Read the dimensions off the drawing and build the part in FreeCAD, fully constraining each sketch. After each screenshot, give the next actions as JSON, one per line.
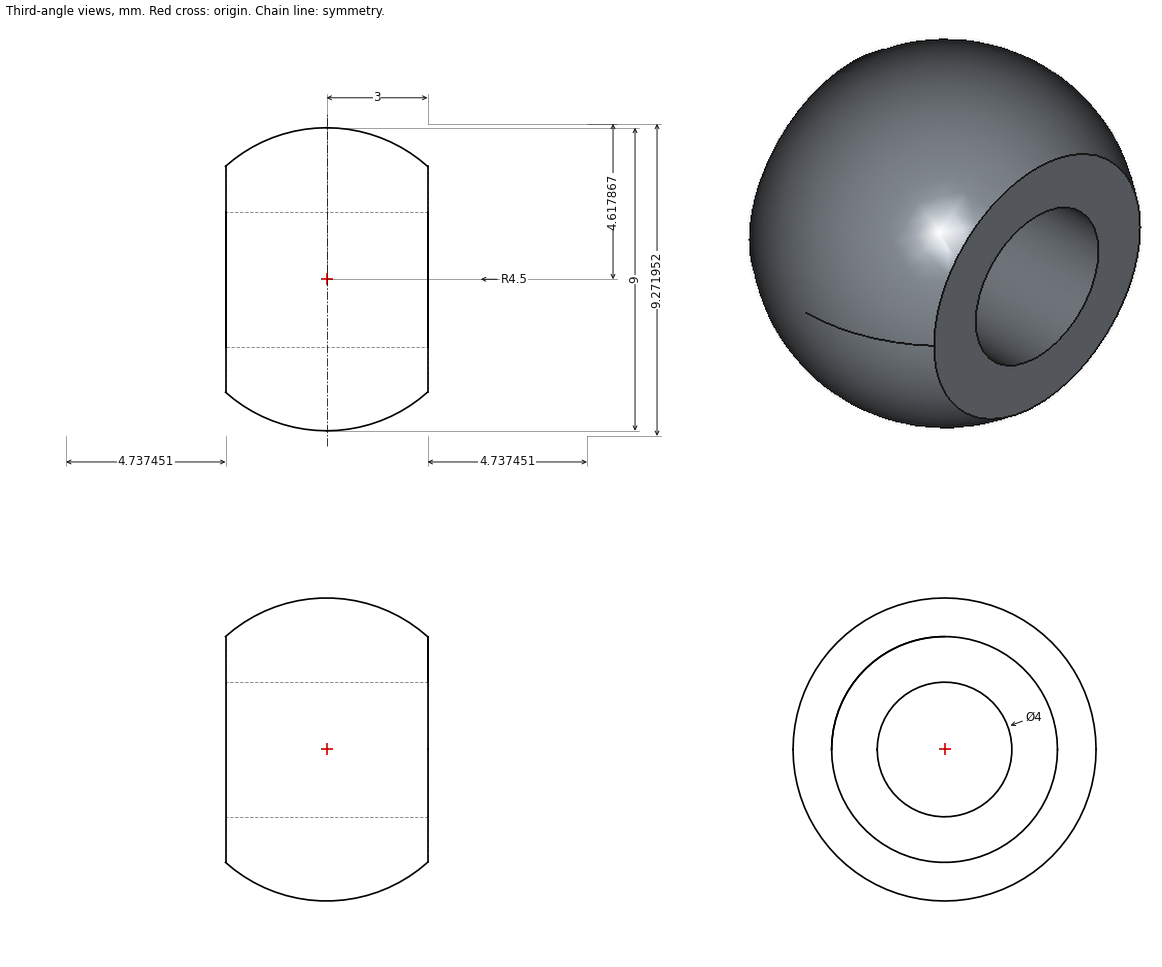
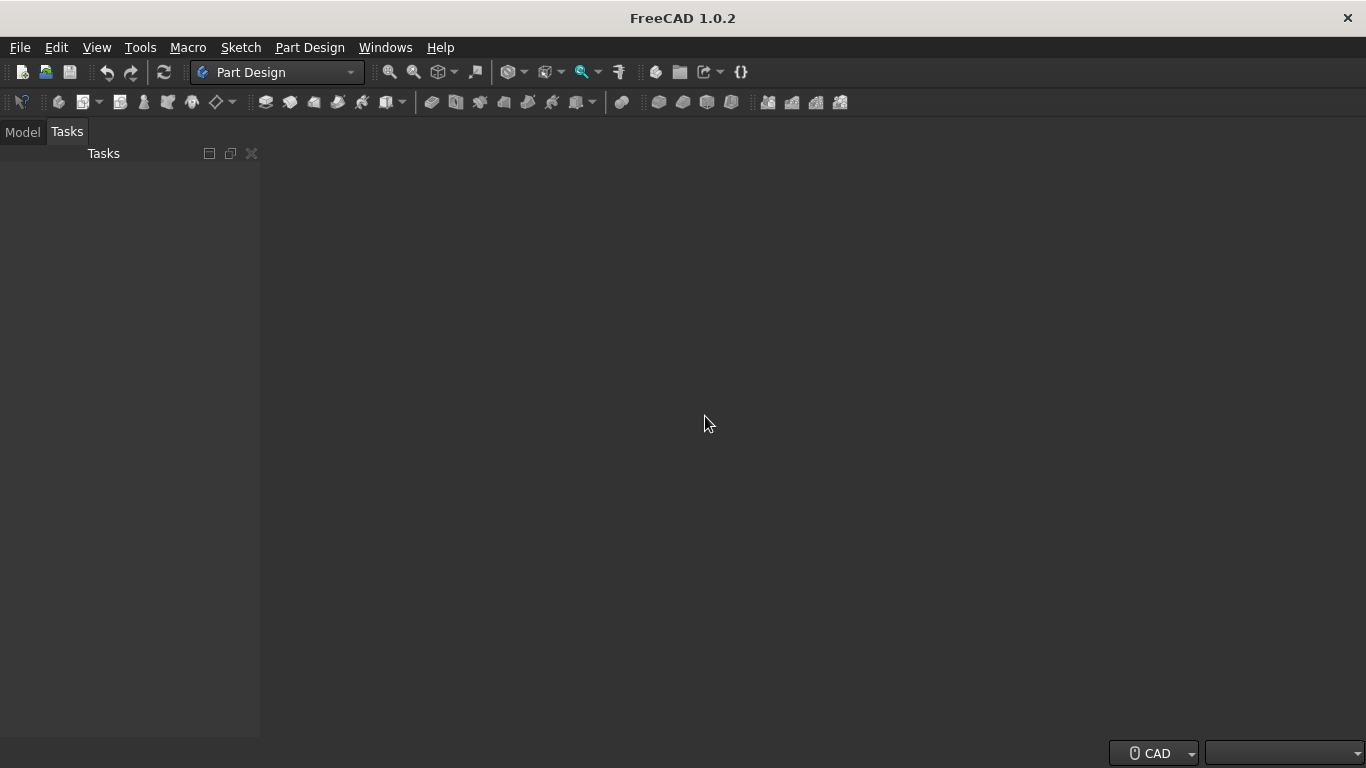
{"action": "left_click", "coordinate": [22, 72]}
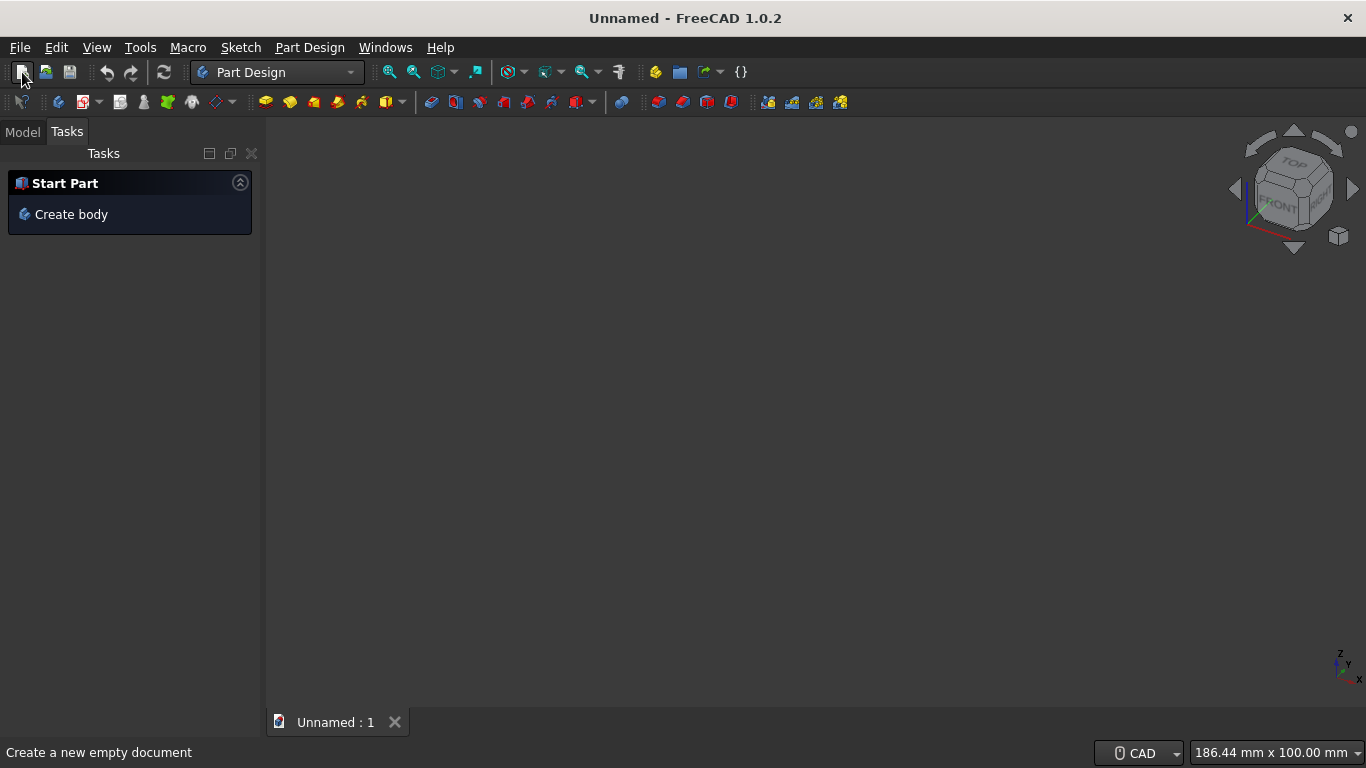
{"action": "left_click", "coordinate": [84, 102]}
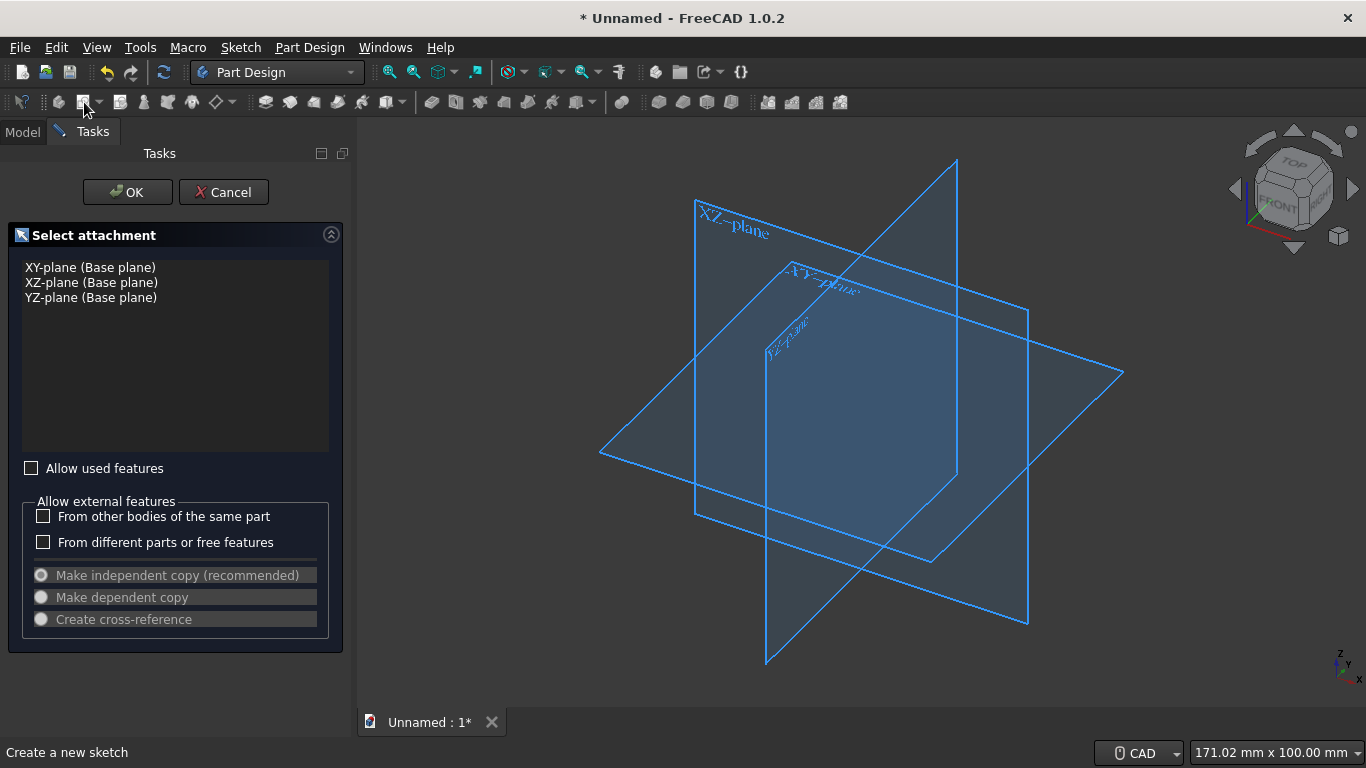
{"action": "left_click", "coordinate": [82, 268]}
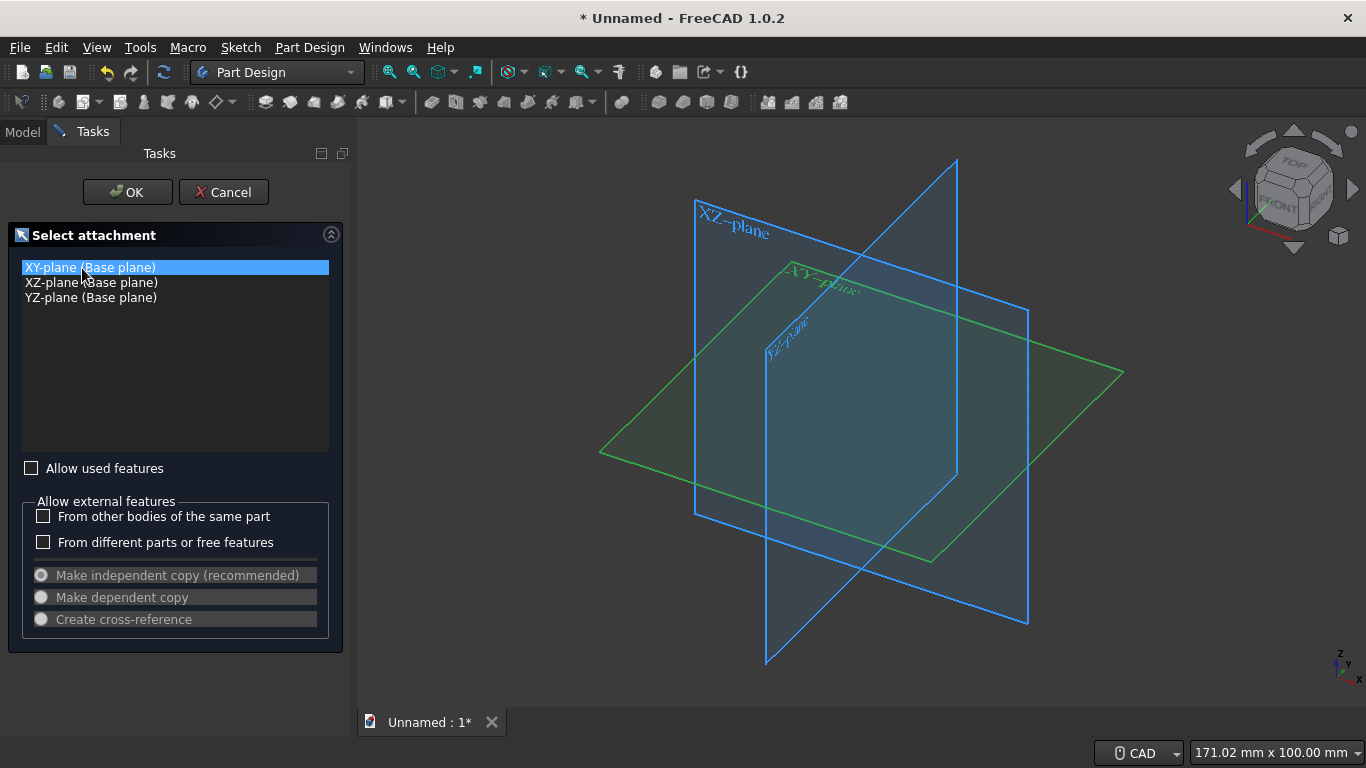
{"action": "left_click", "coordinate": [128, 192]}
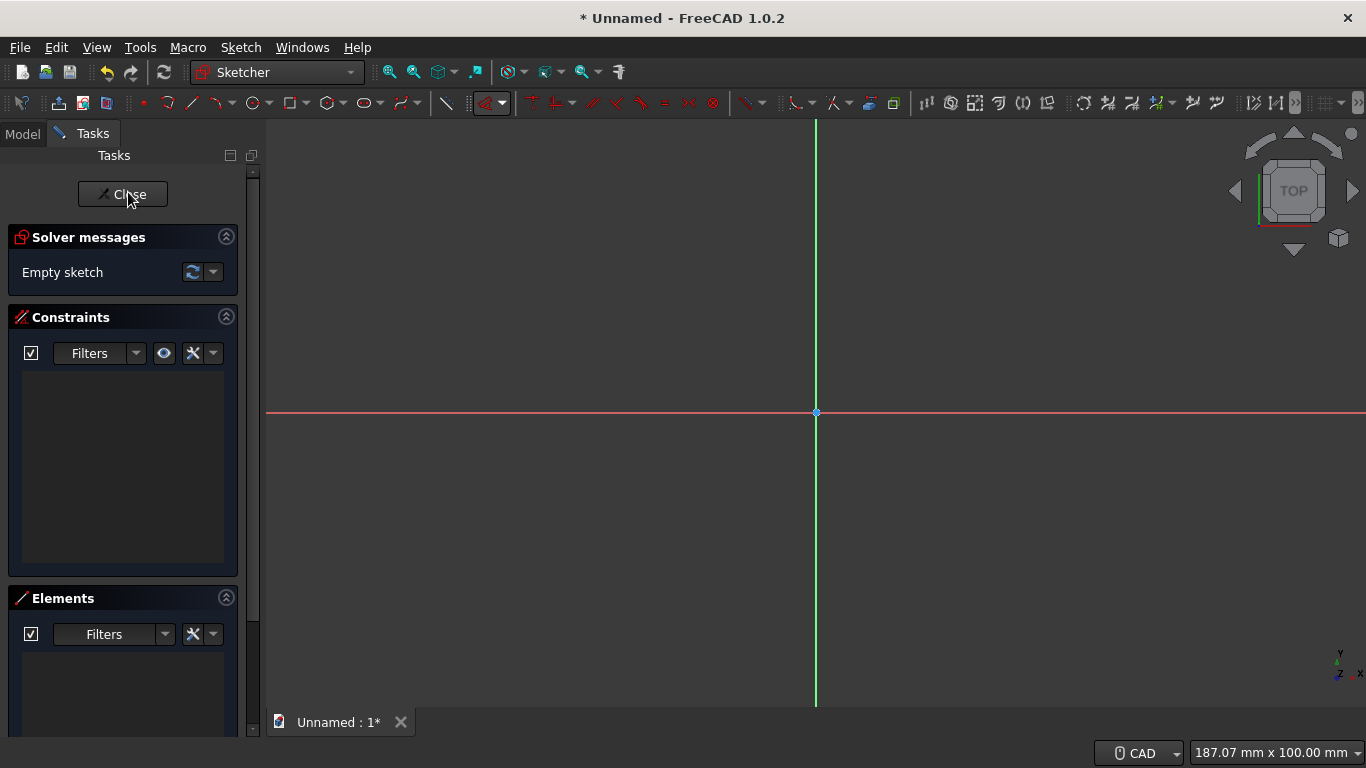
{"action": "scroll", "coordinate": [842, 413], "scroll_direction": "up", "scroll_amount": 10}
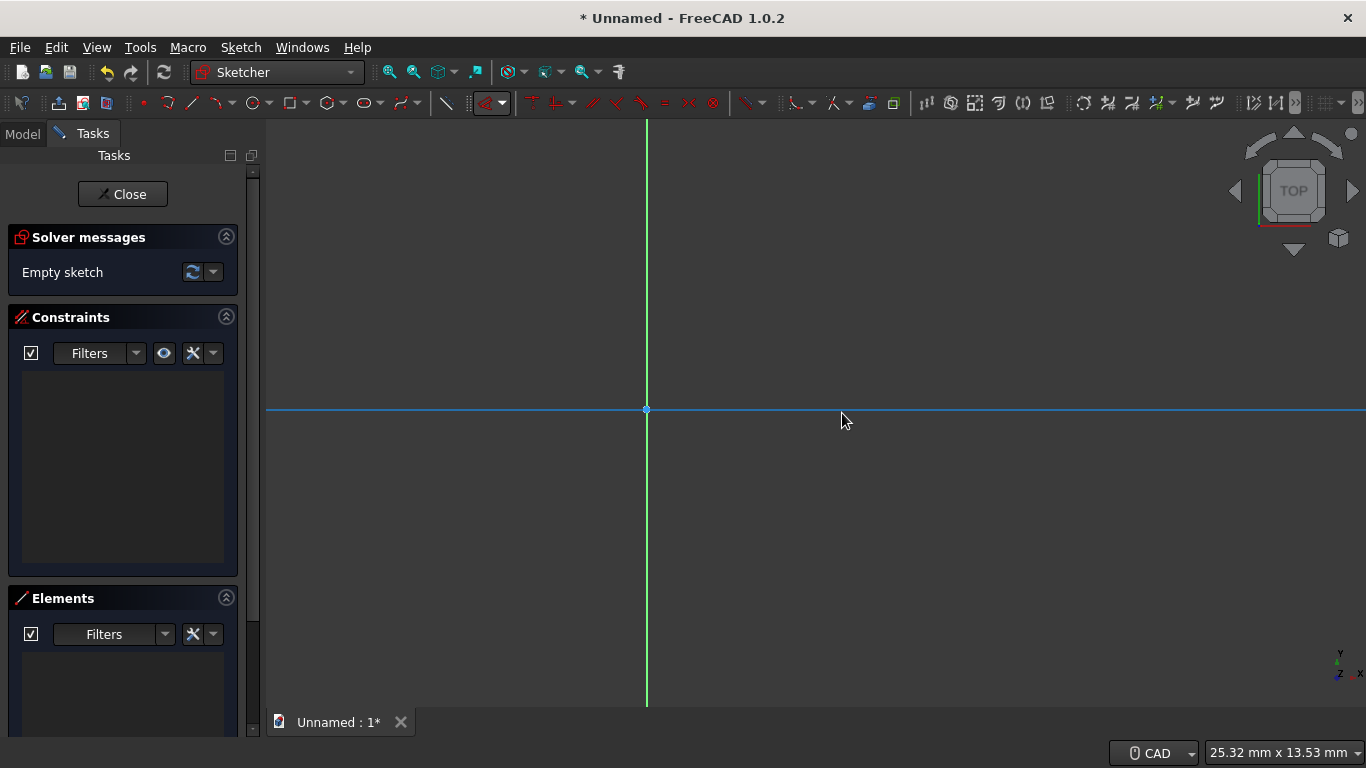
{"action": "left_click", "coordinate": [192, 104]}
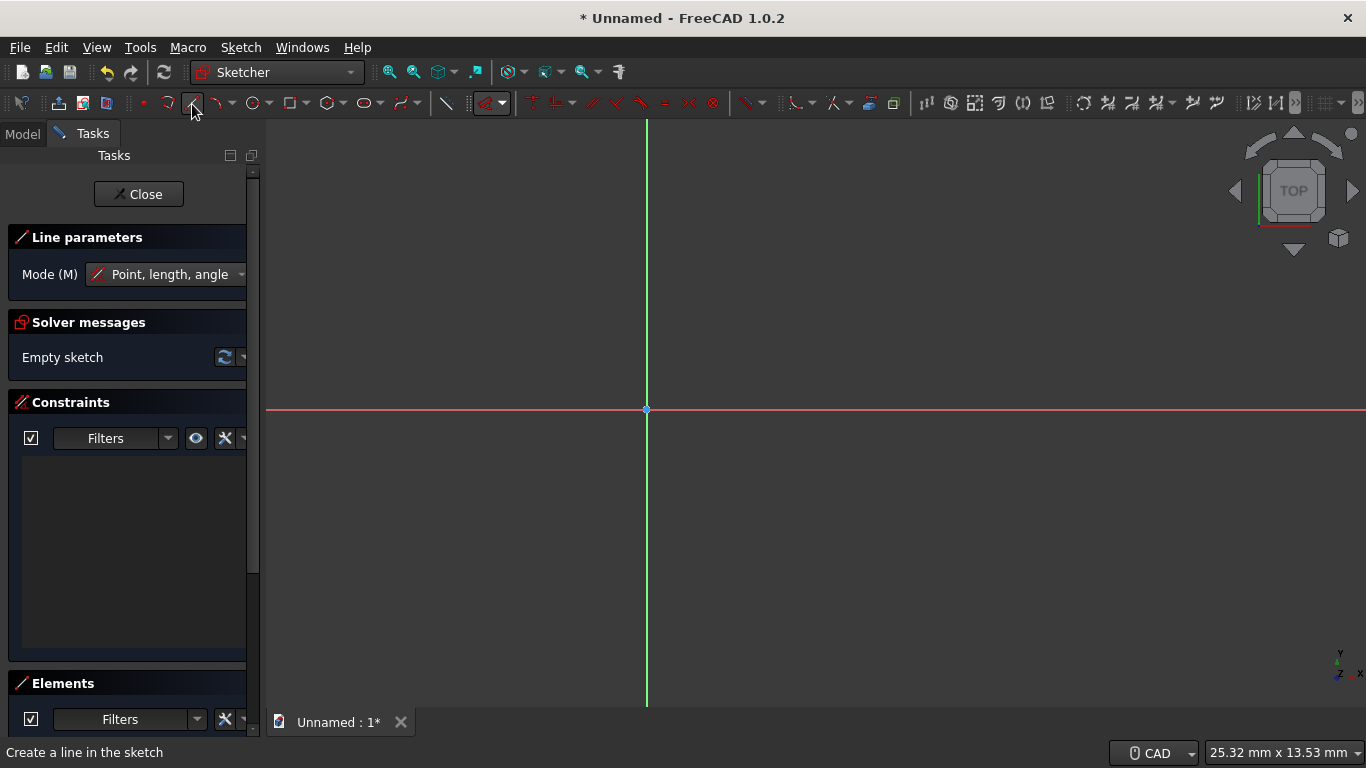
{"action": "left_click", "coordinate": [647, 214]}
{"action": "left_click", "coordinate": [656, 605]}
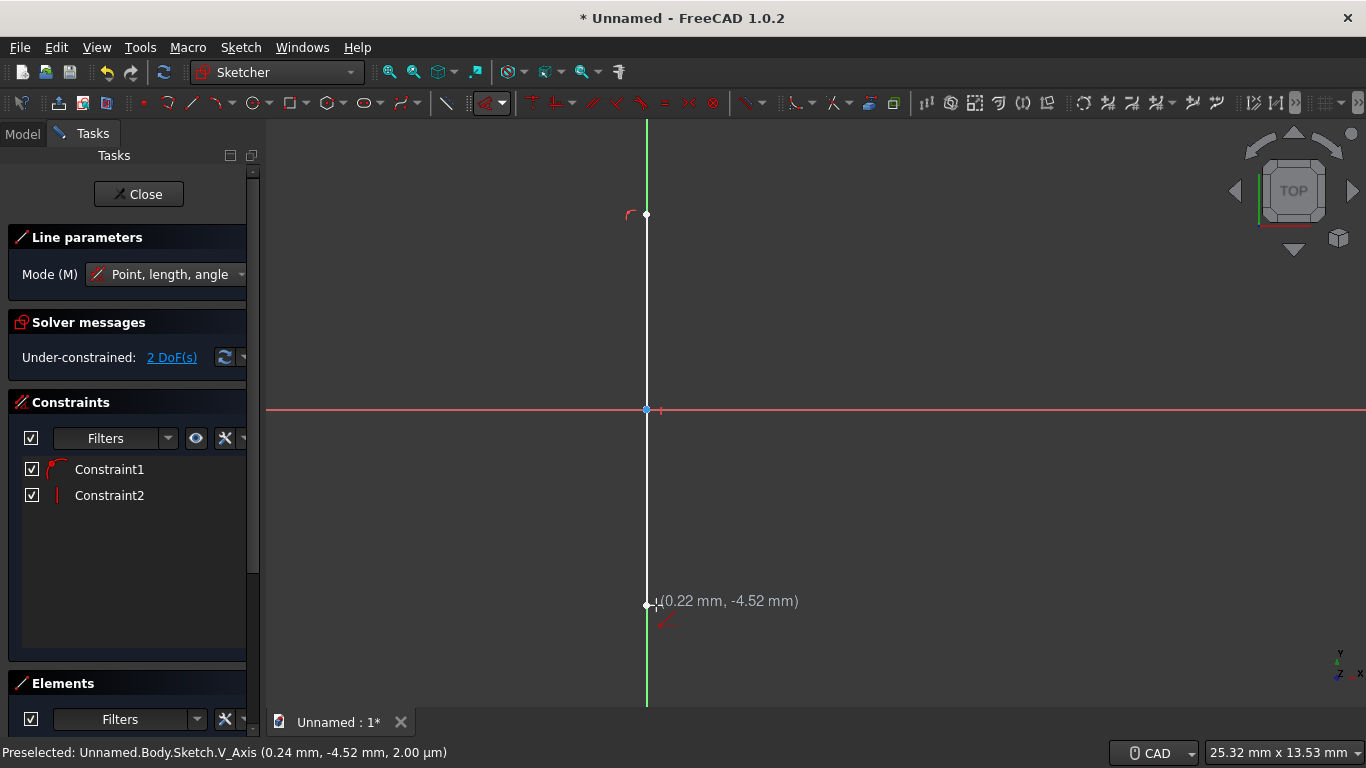
{"action": "key", "text": "g 3 a"}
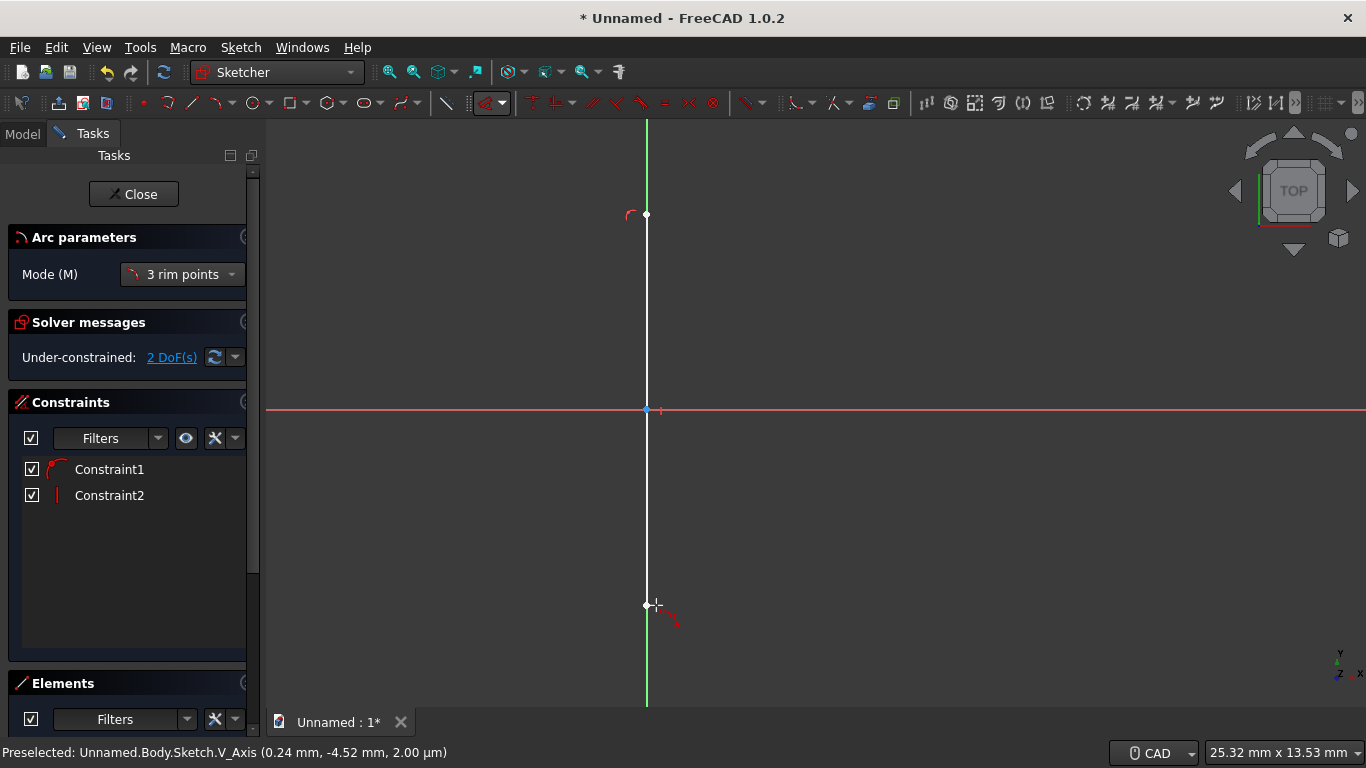
{"action": "left_click", "coordinate": [656, 605]}
{"action": "left_click", "coordinate": [647, 215]}
{"action": "left_click", "coordinate": [832, 470]}
{"action": "key", "text": "Escape"}